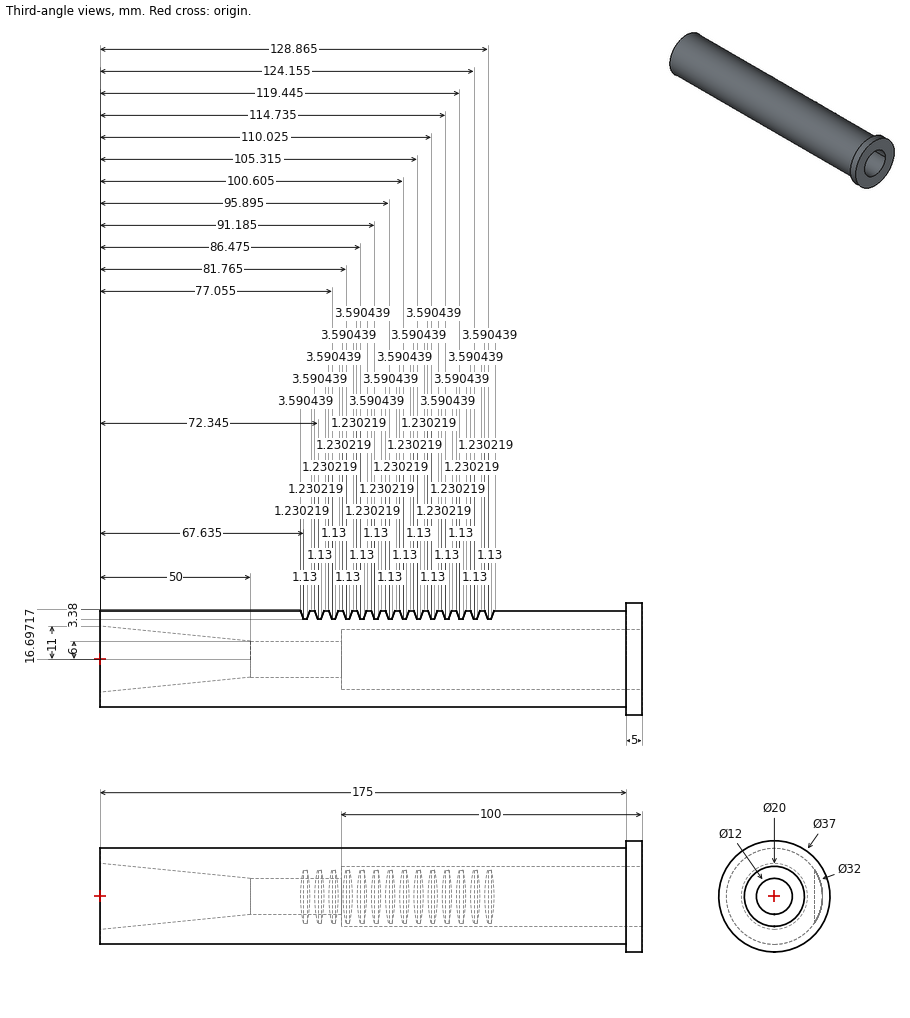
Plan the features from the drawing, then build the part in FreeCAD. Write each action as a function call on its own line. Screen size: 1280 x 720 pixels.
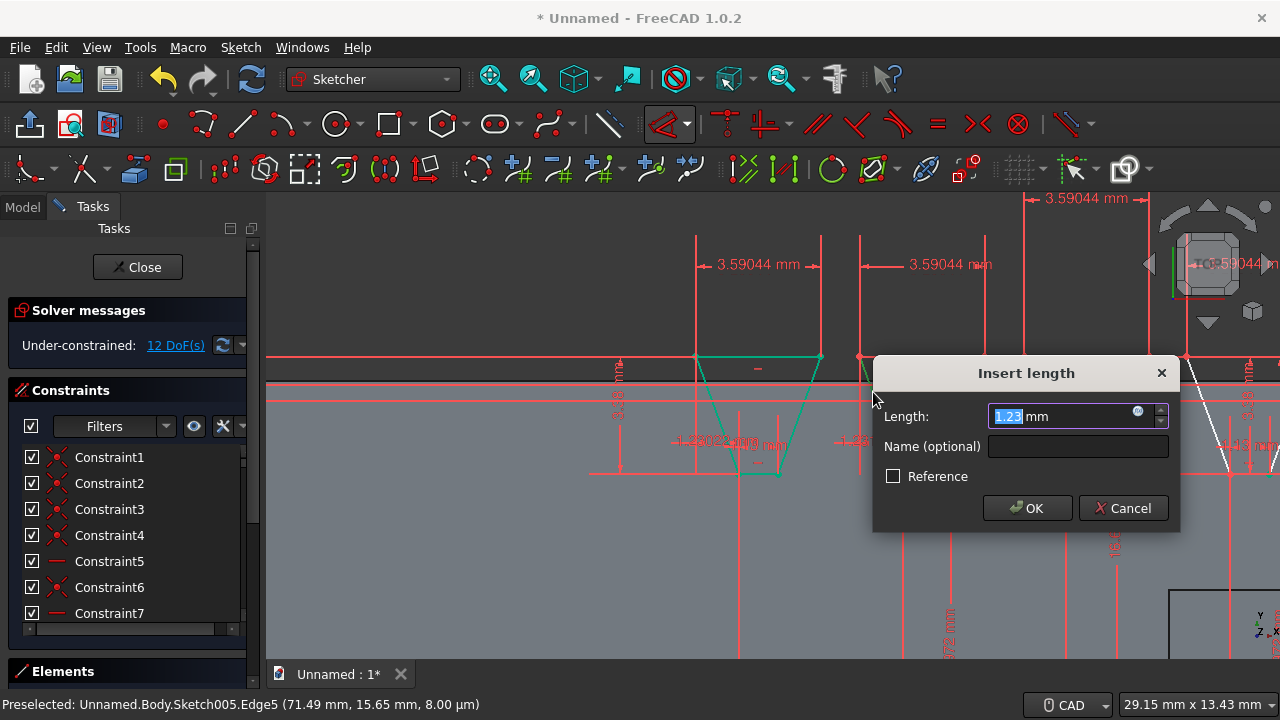
text(1.230219)
key(Return)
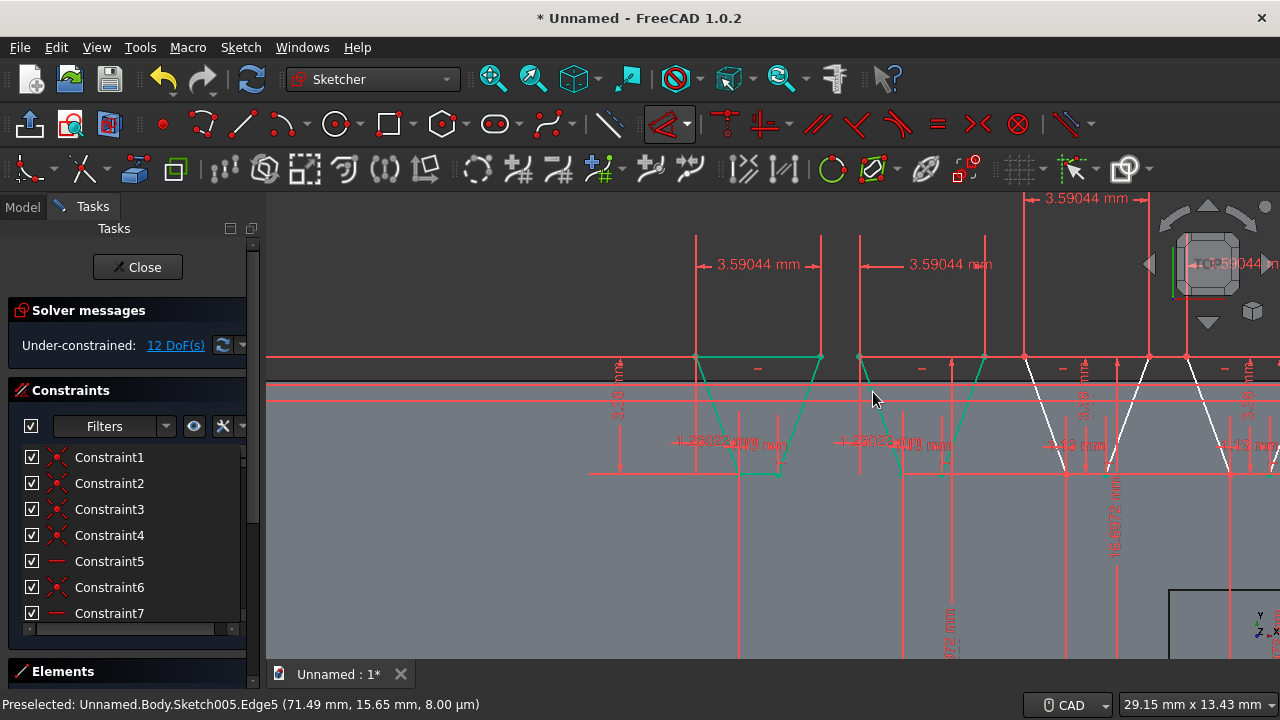
click(1037, 392)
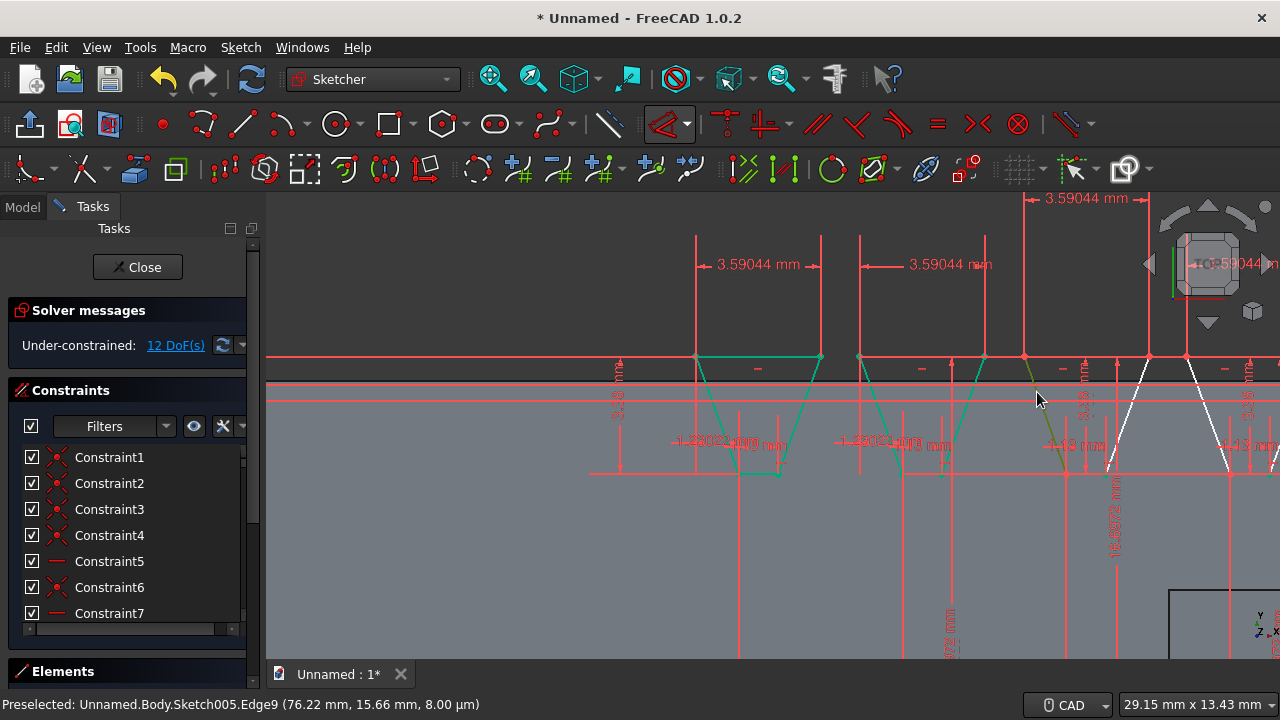
key(l)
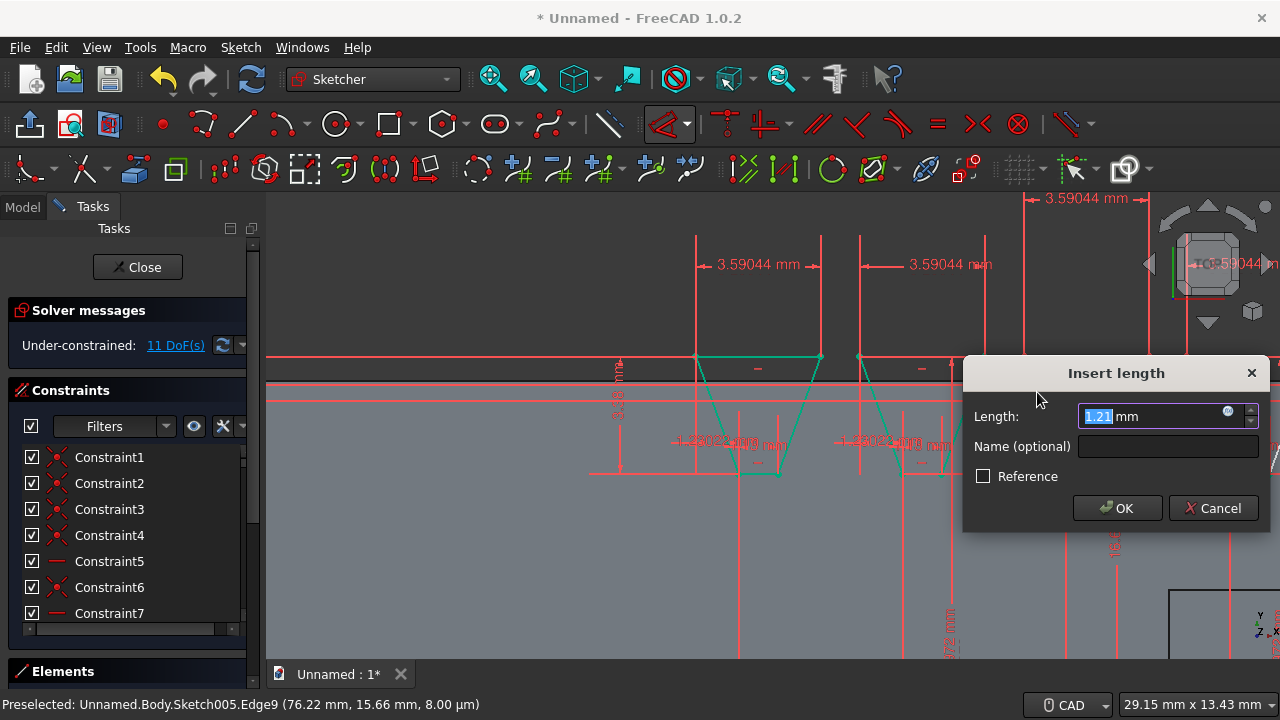
text(1.230219)
key(Return)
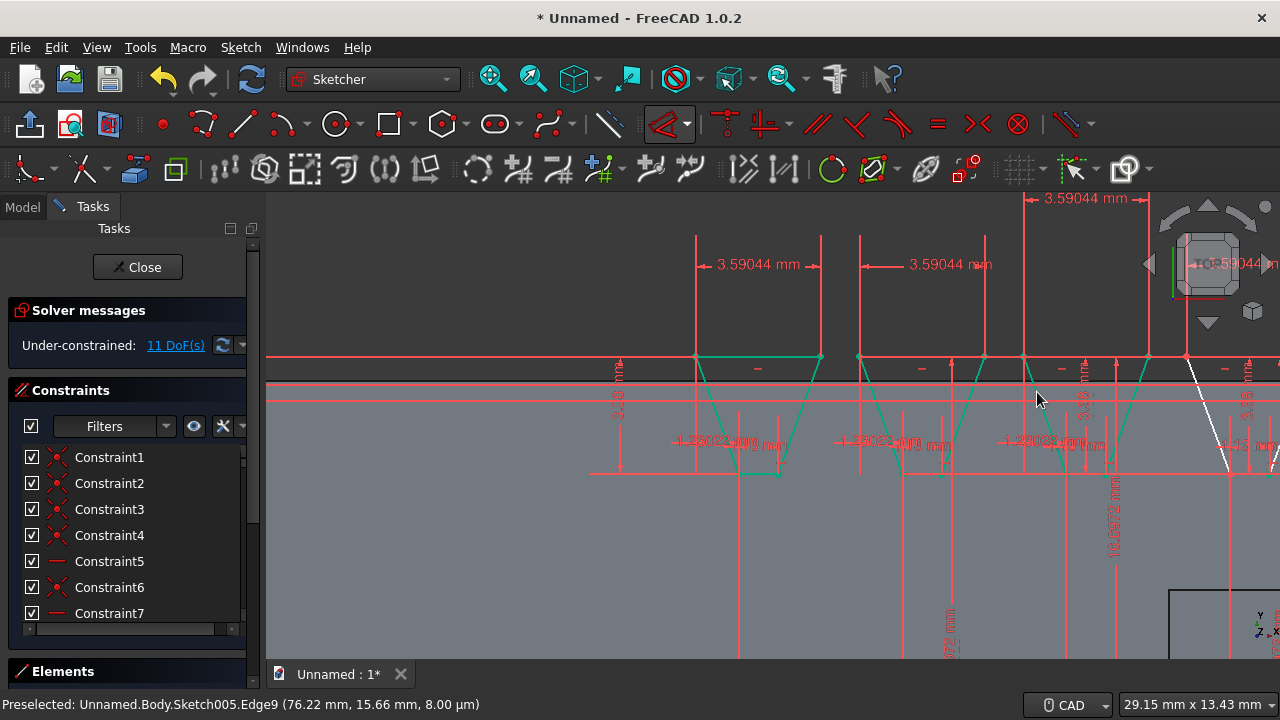
scroll(710, 391, down, 10)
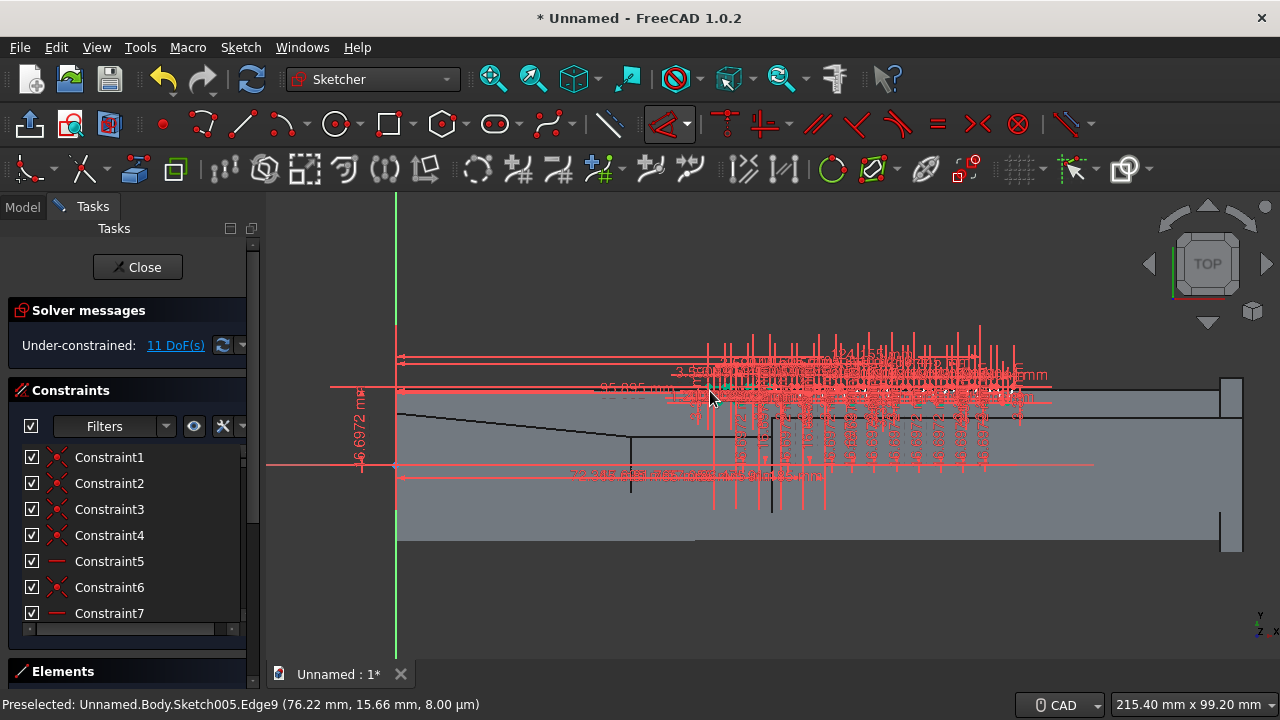
scroll(777, 391, up, 10)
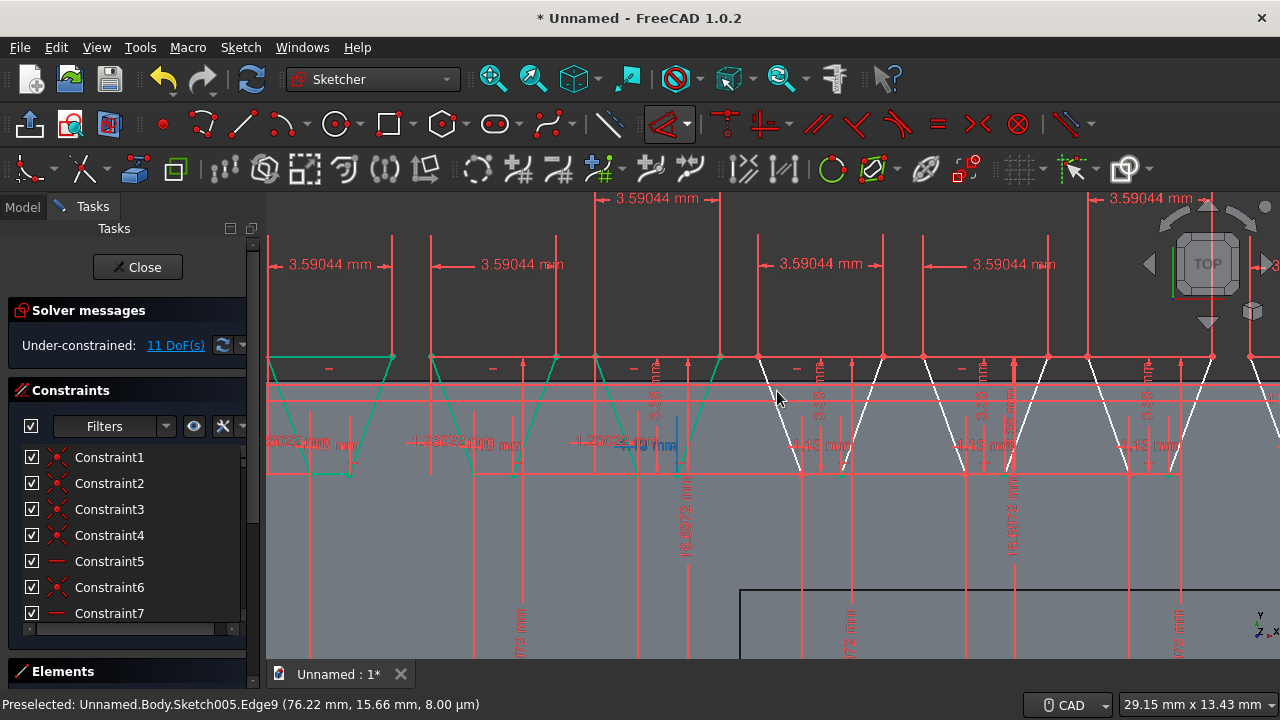
click(771, 392)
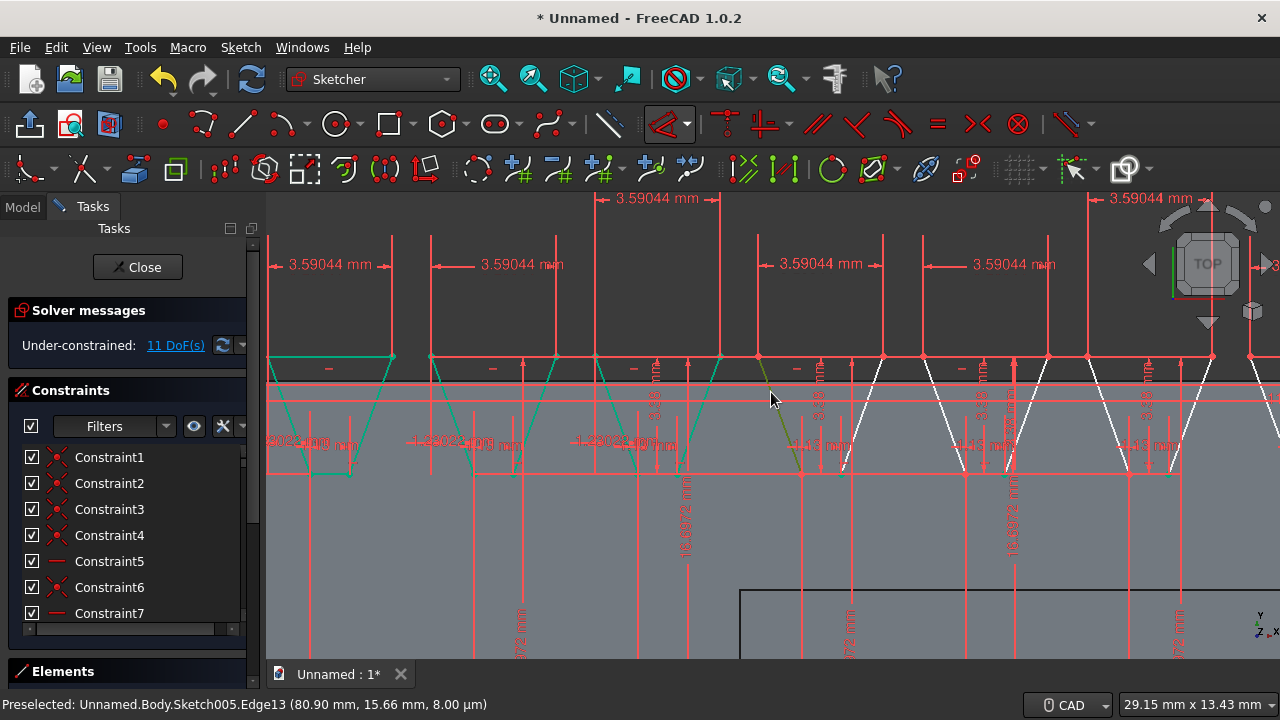
key(l)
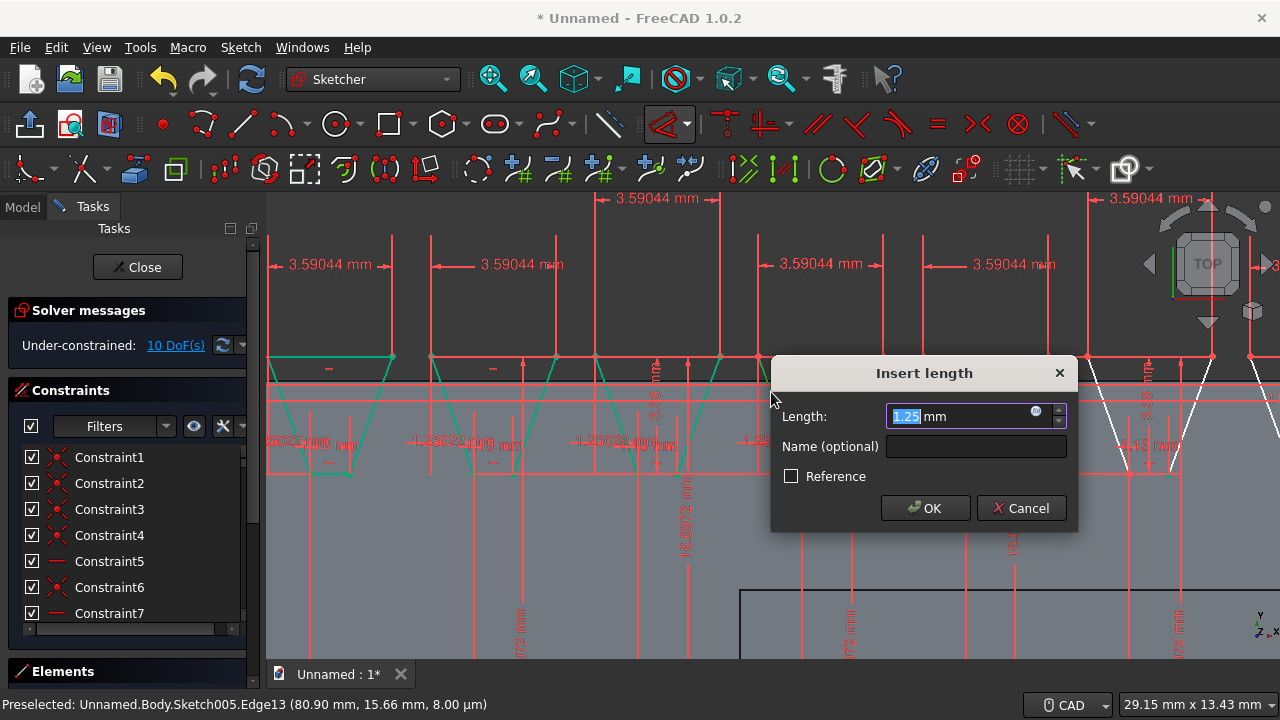
text(1.230219)
key(Return)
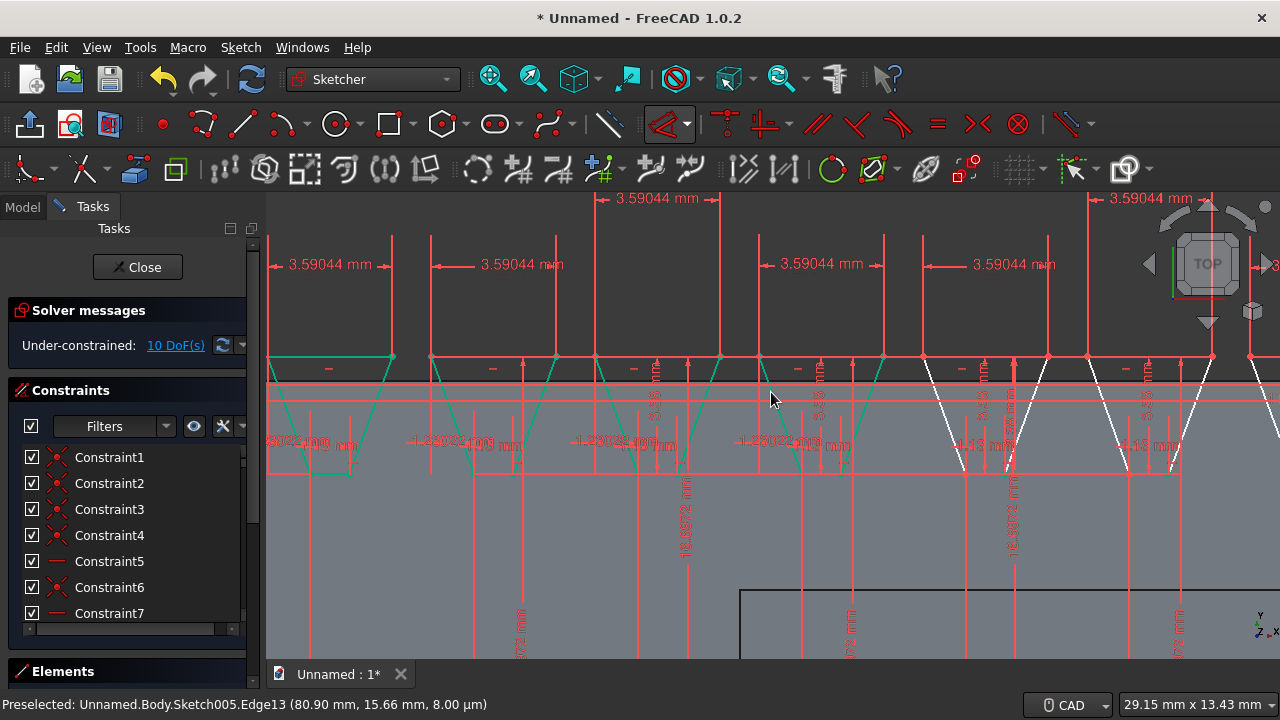
click(936, 392)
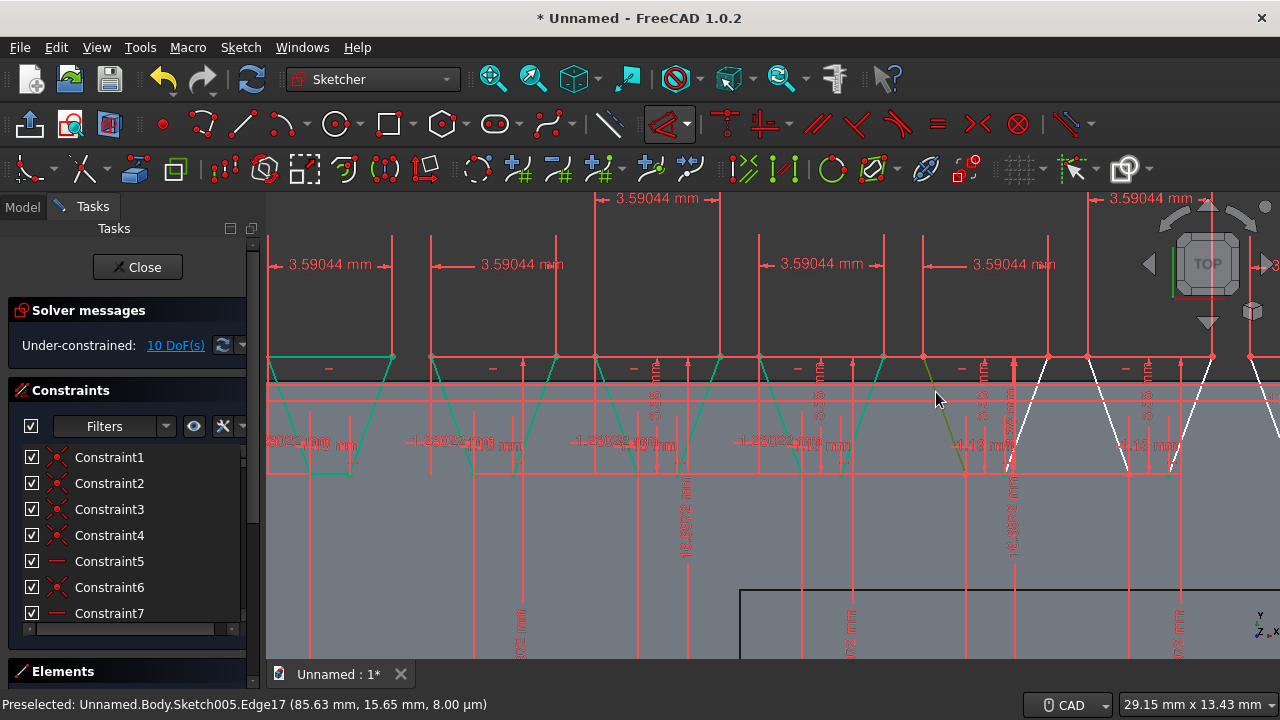
key(l)